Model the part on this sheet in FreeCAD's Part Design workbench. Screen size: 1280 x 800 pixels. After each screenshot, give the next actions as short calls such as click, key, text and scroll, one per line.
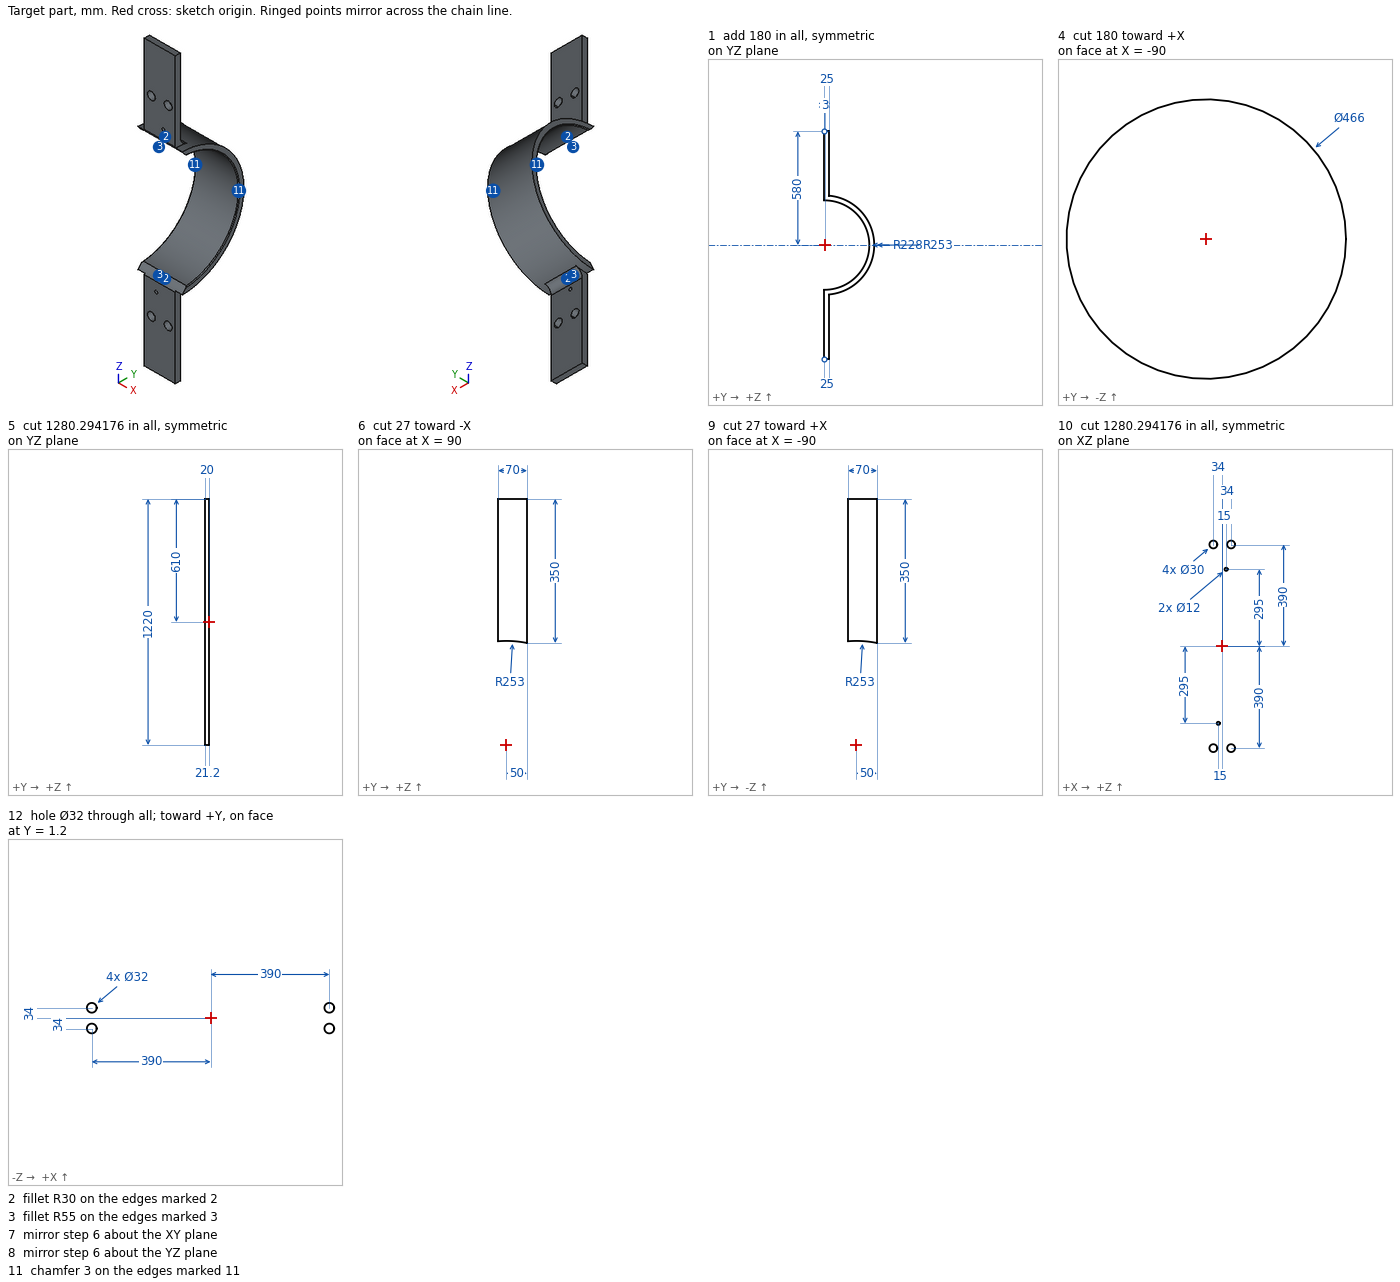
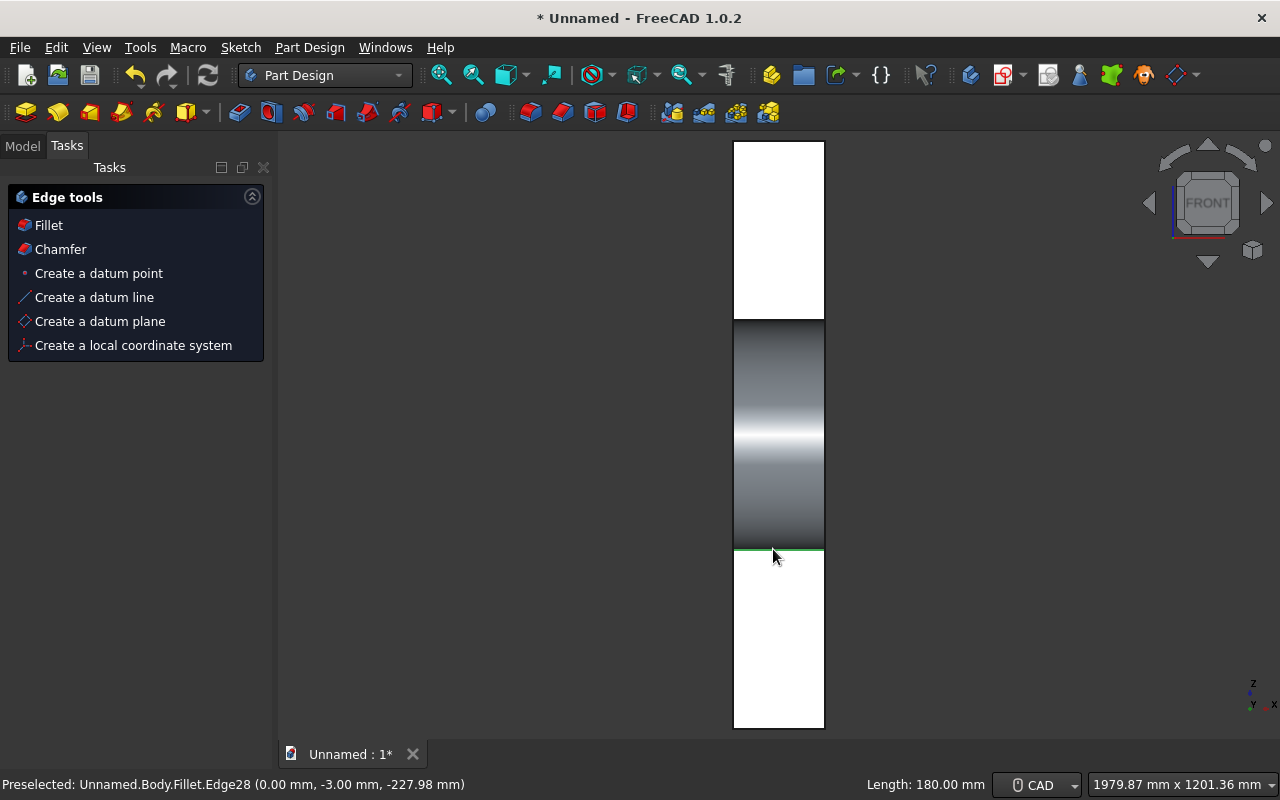
click(779, 319, ctrl)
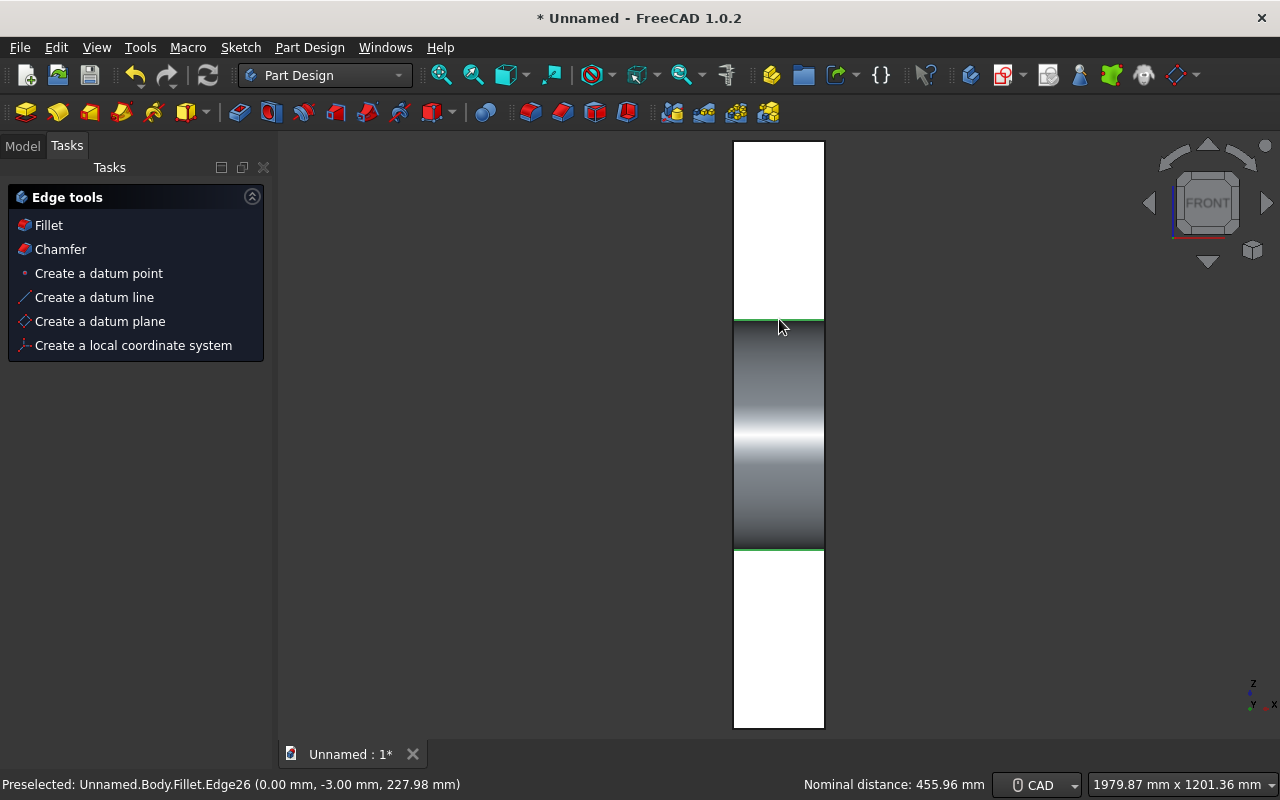
click(532, 112)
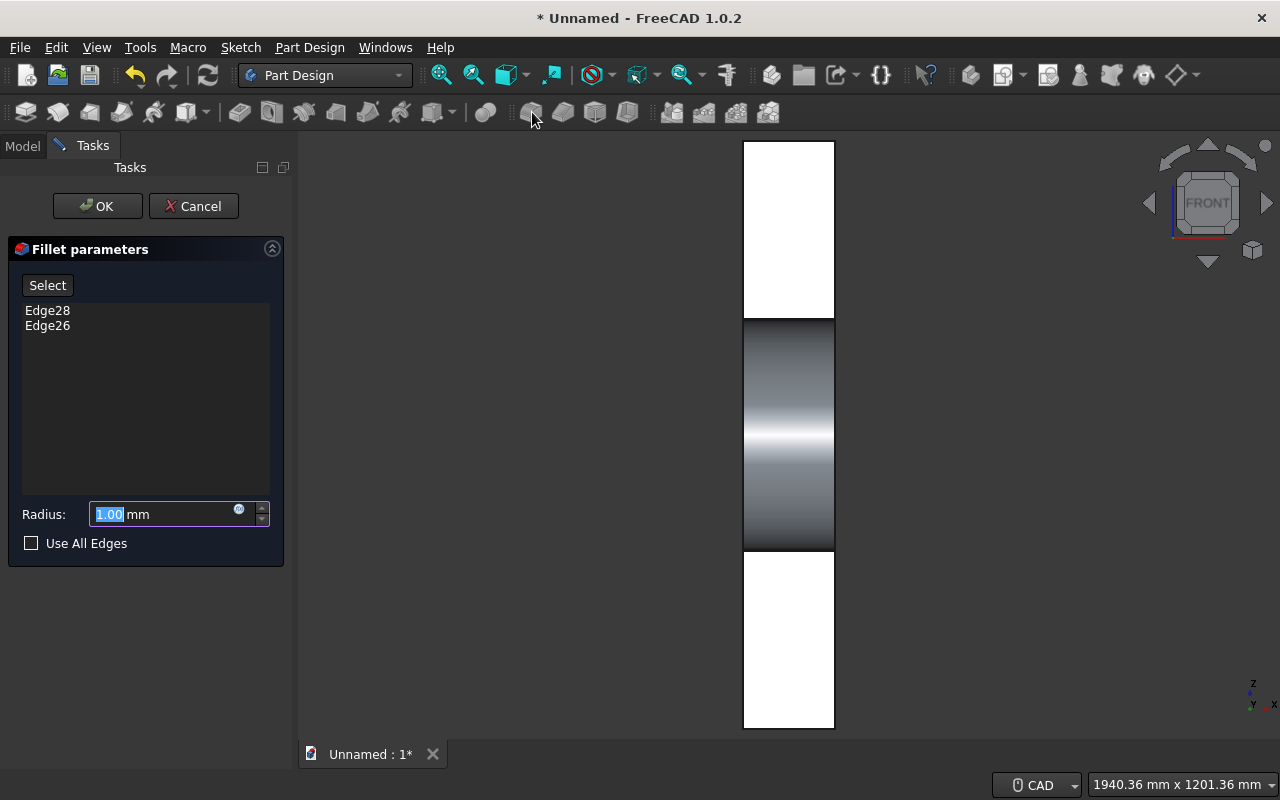
text(55)
key(Tab)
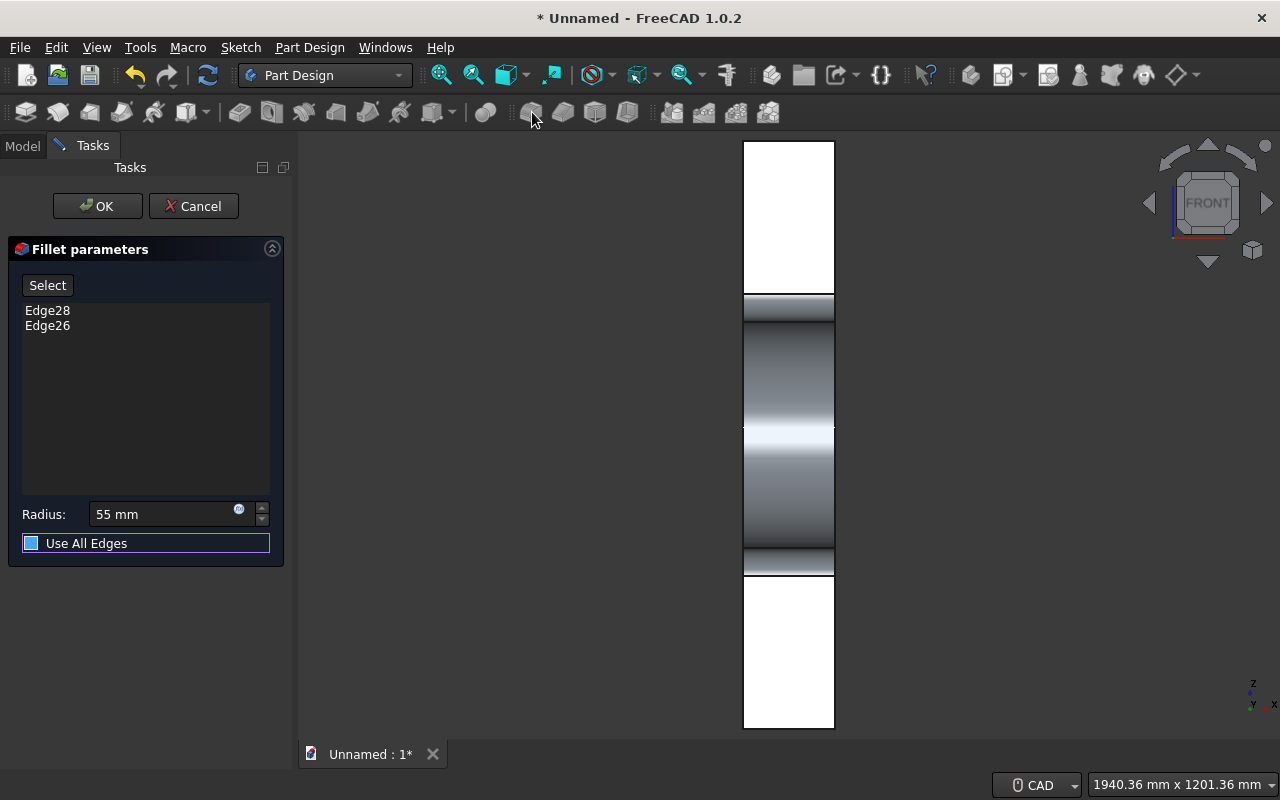
click(98, 206)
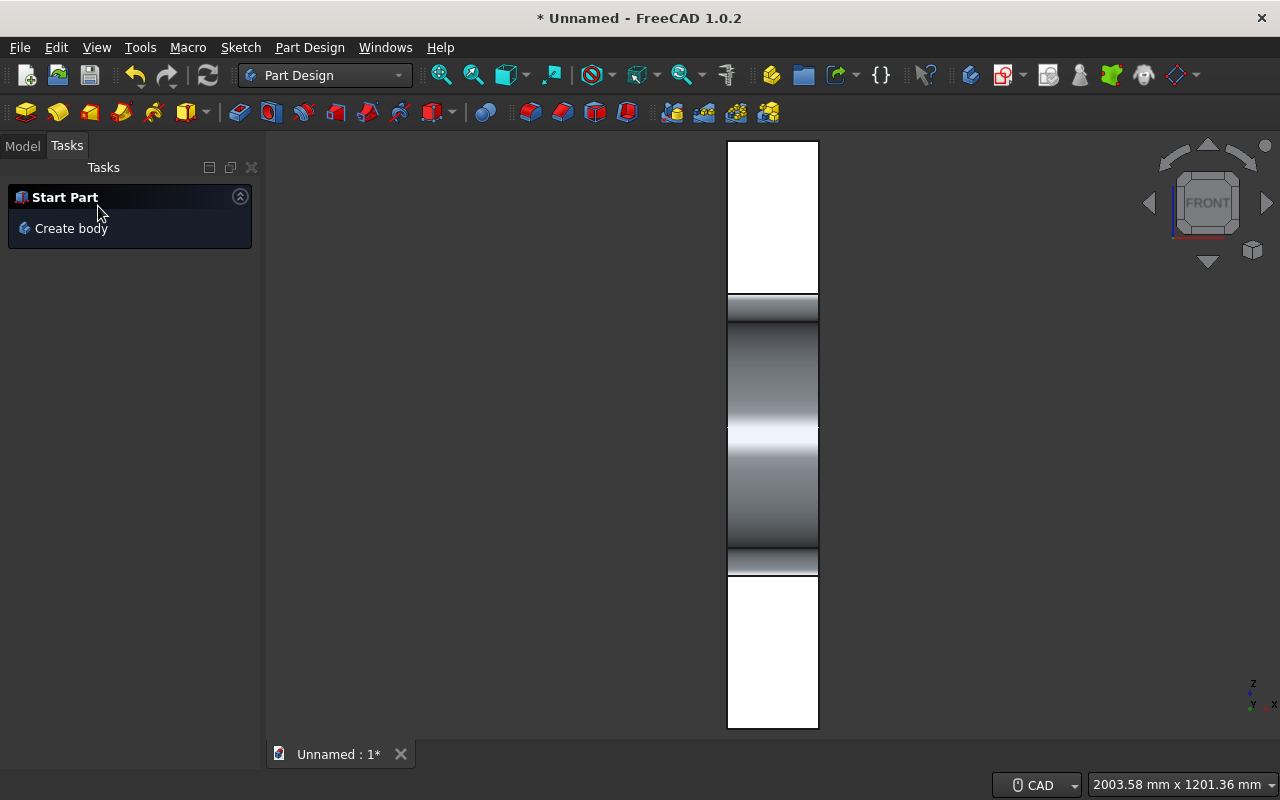
key(6)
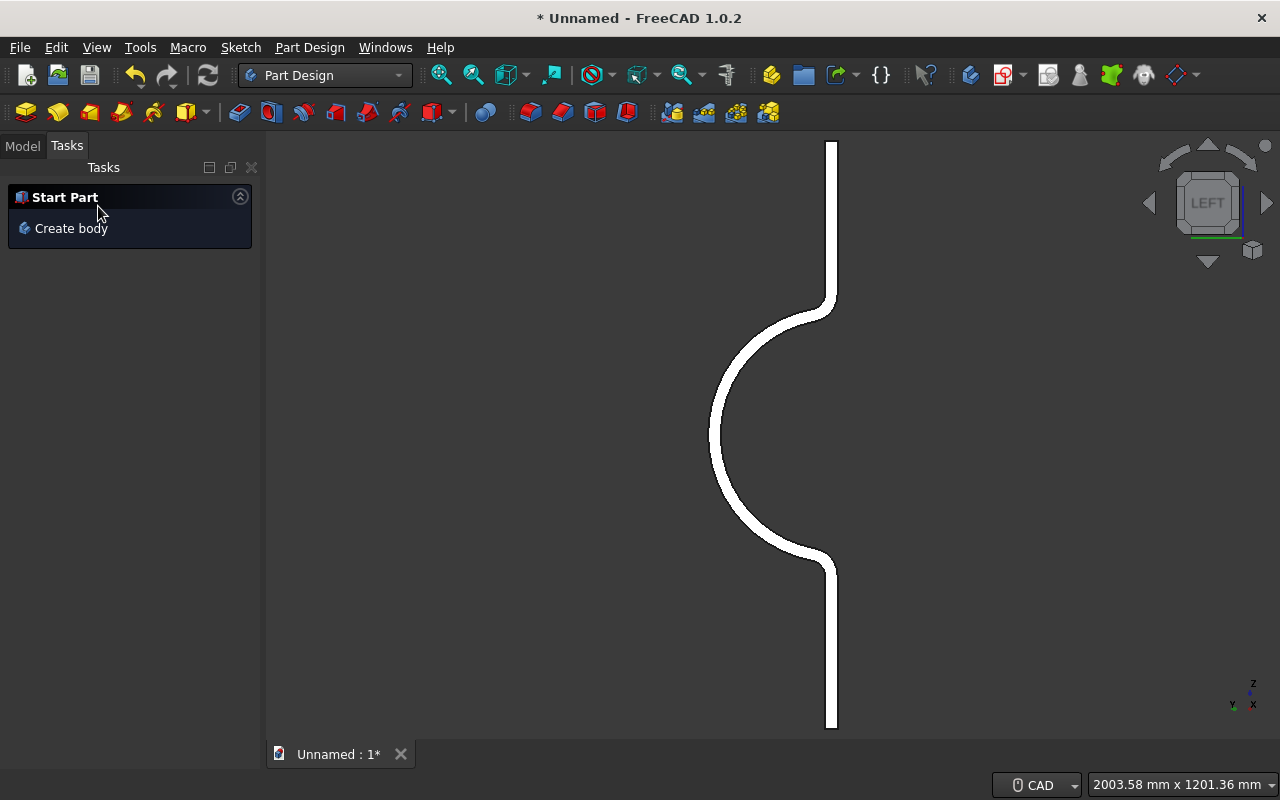
scroll(828, 182, up, 7)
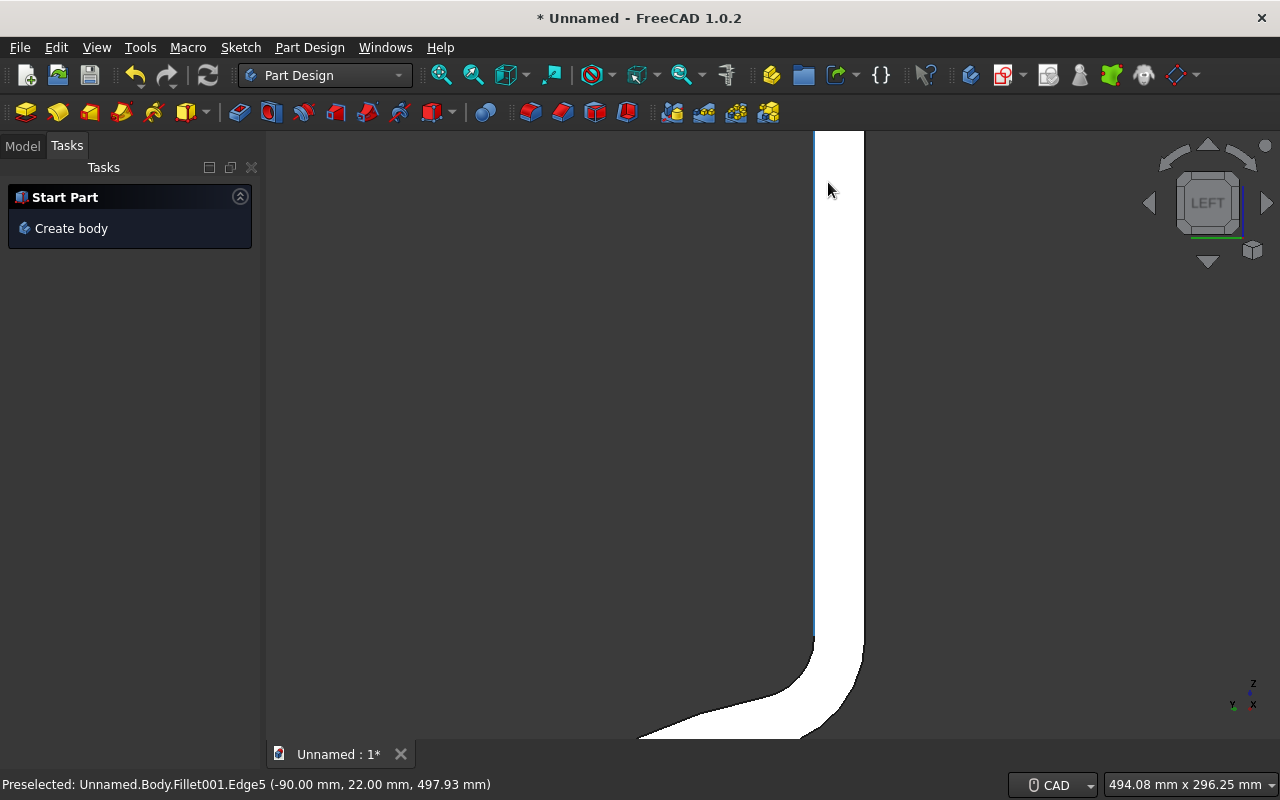
click(828, 186)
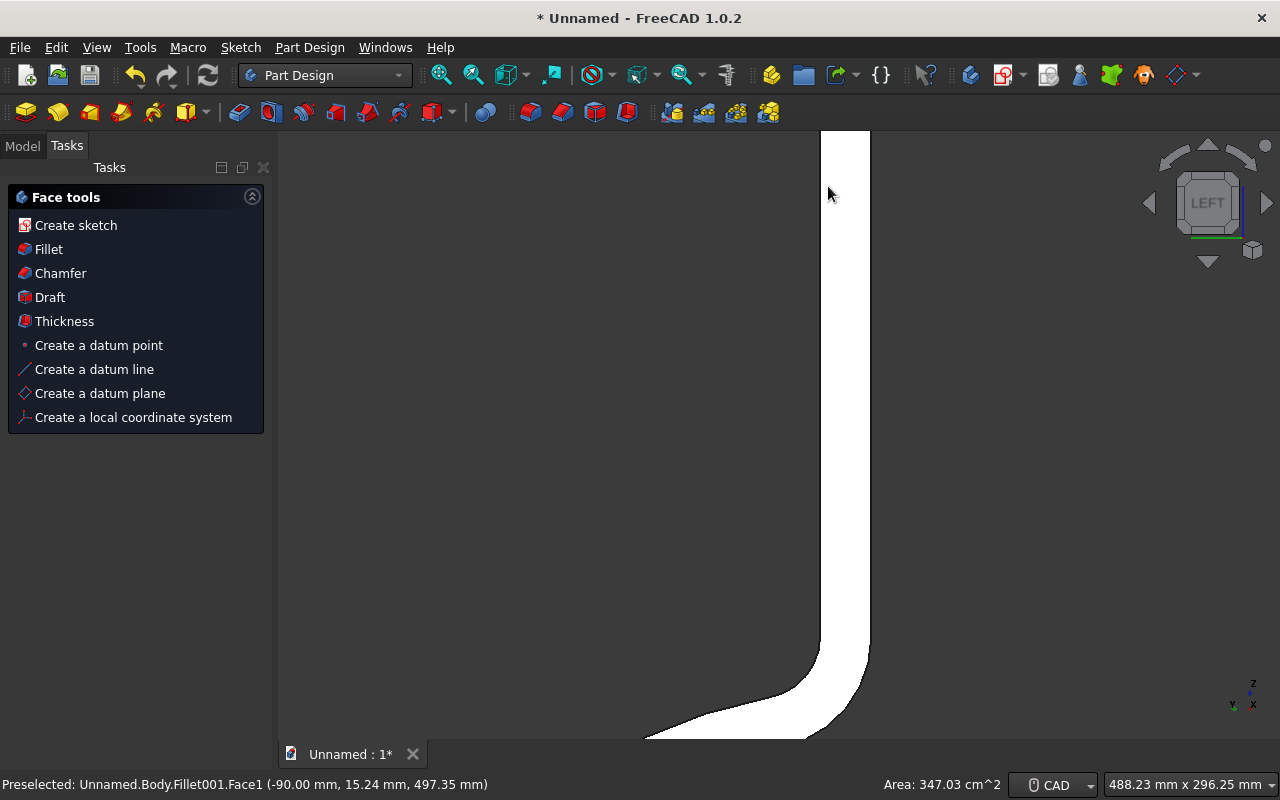
click(1004, 76)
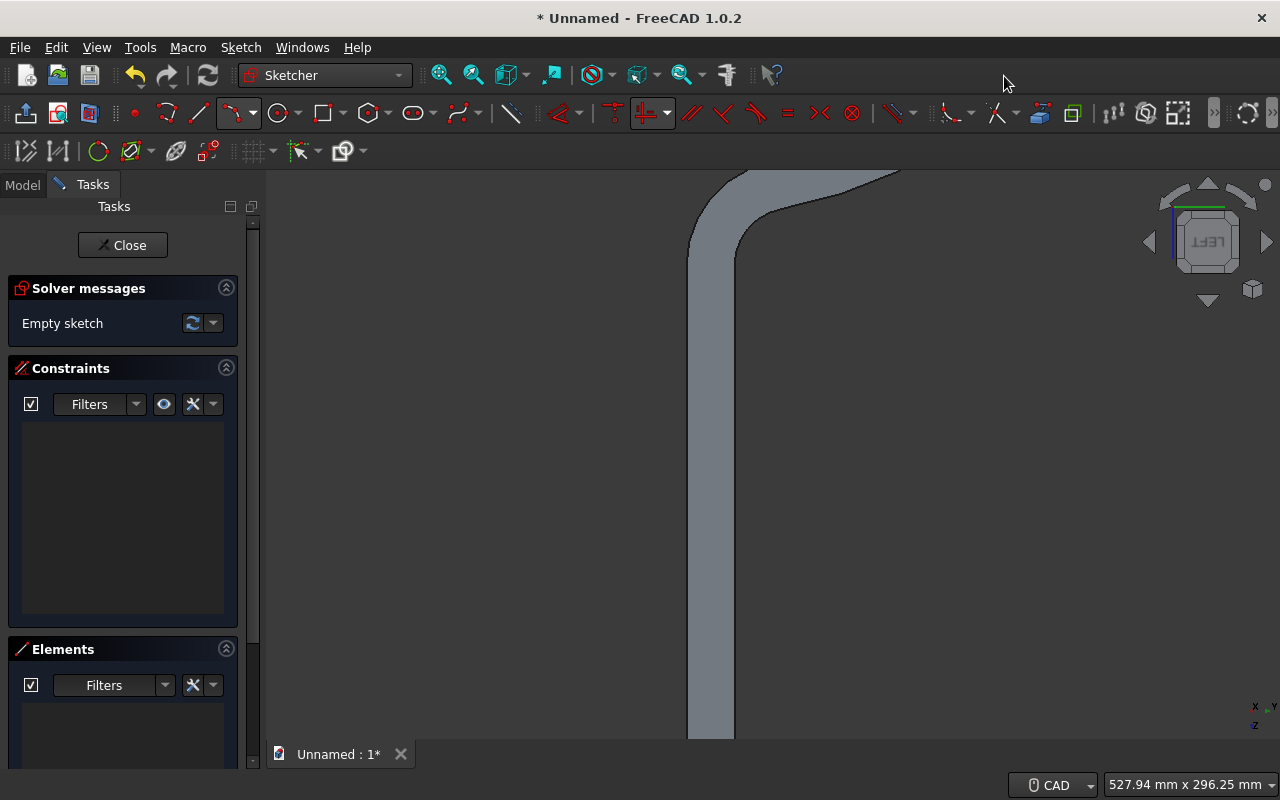
scroll(710, 711, down, 6)